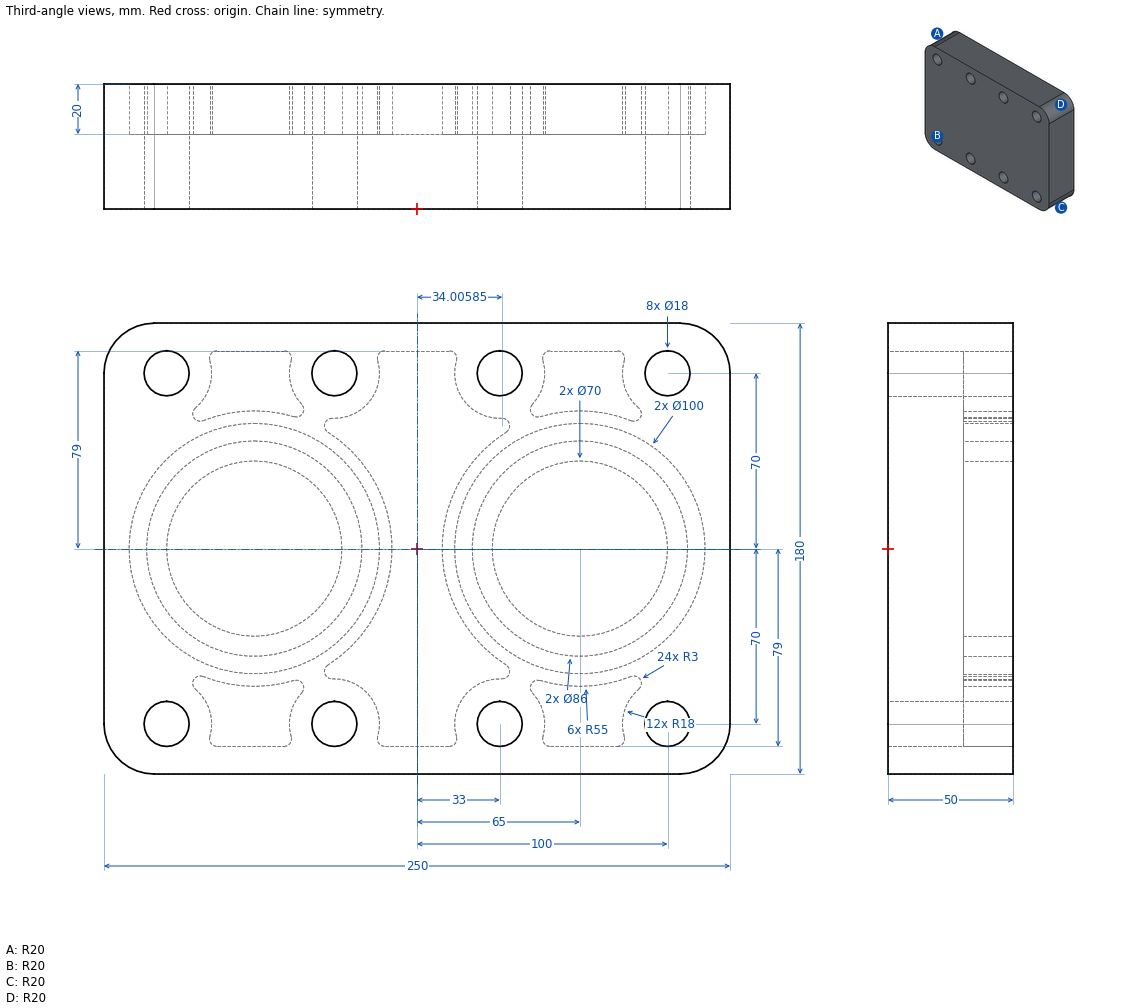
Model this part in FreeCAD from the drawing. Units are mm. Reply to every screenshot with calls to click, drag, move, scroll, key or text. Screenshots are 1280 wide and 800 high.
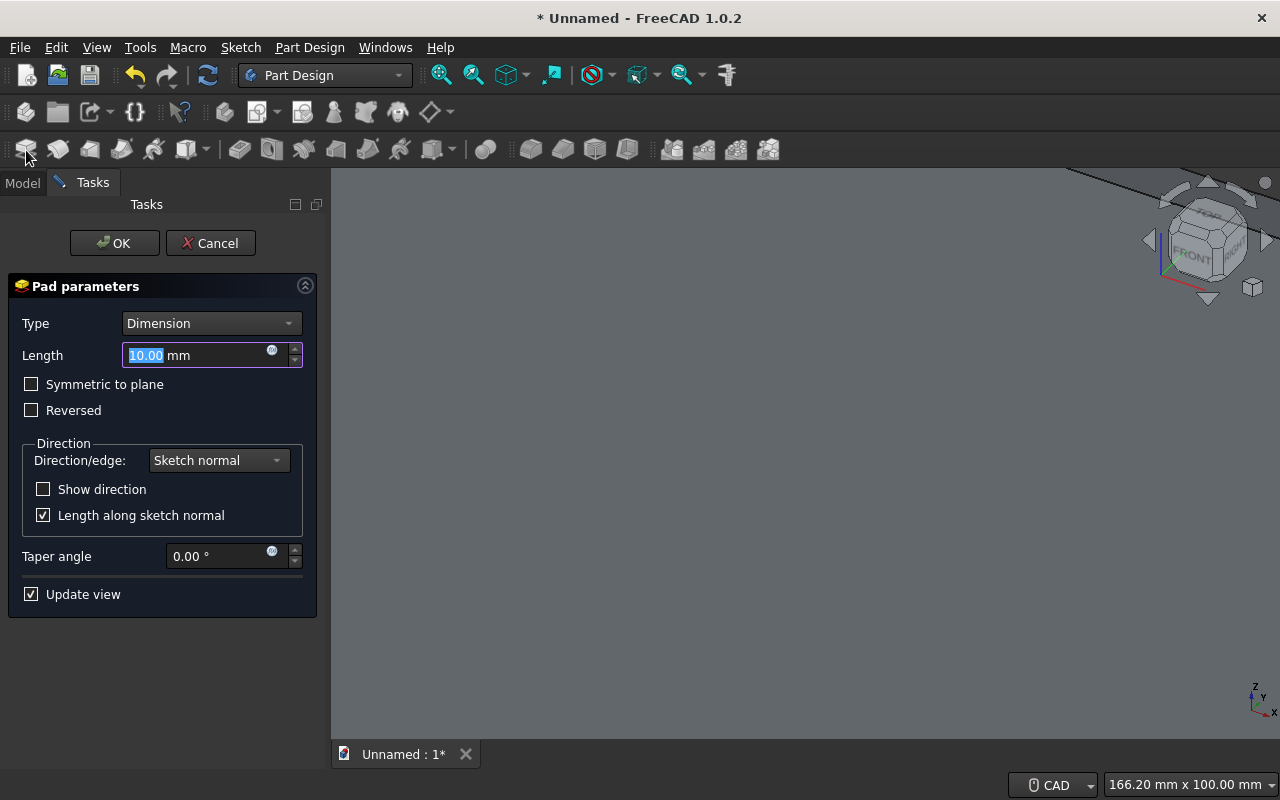
text(50)
key(Tab)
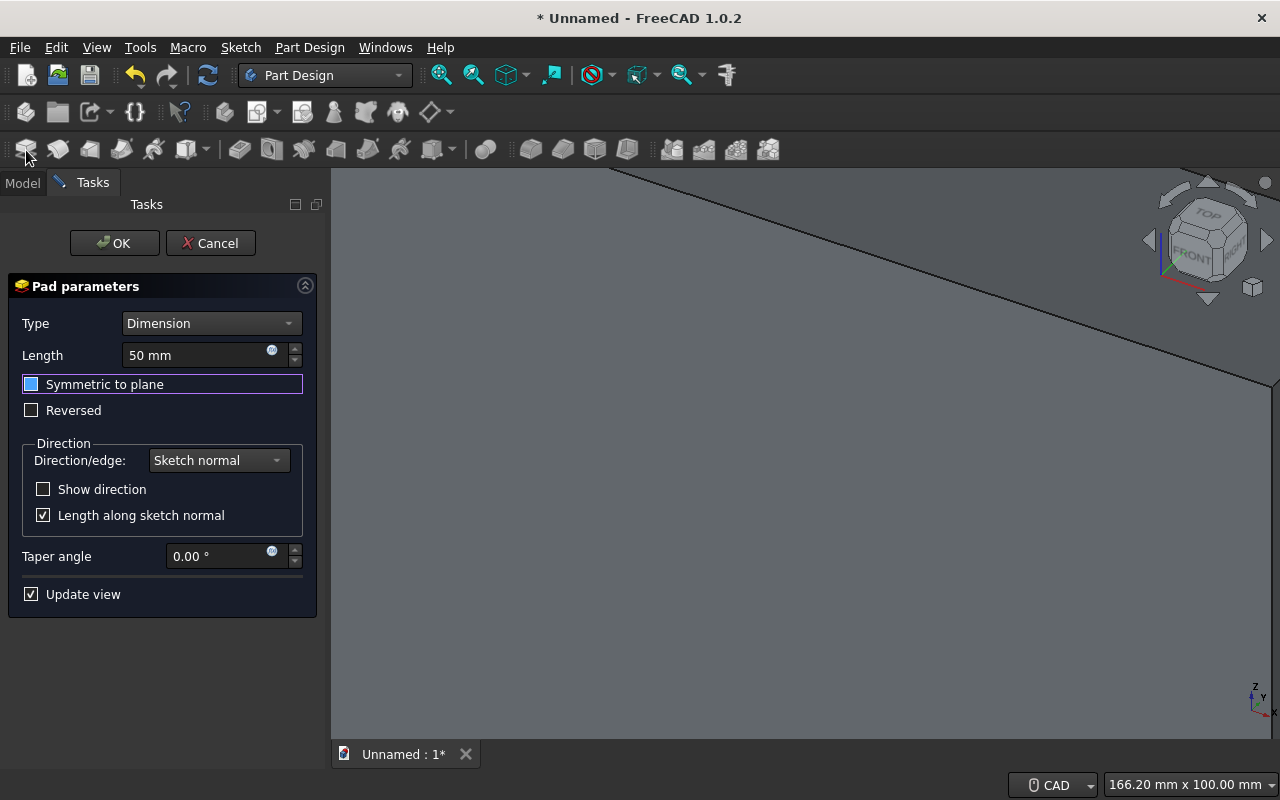
click(30, 410)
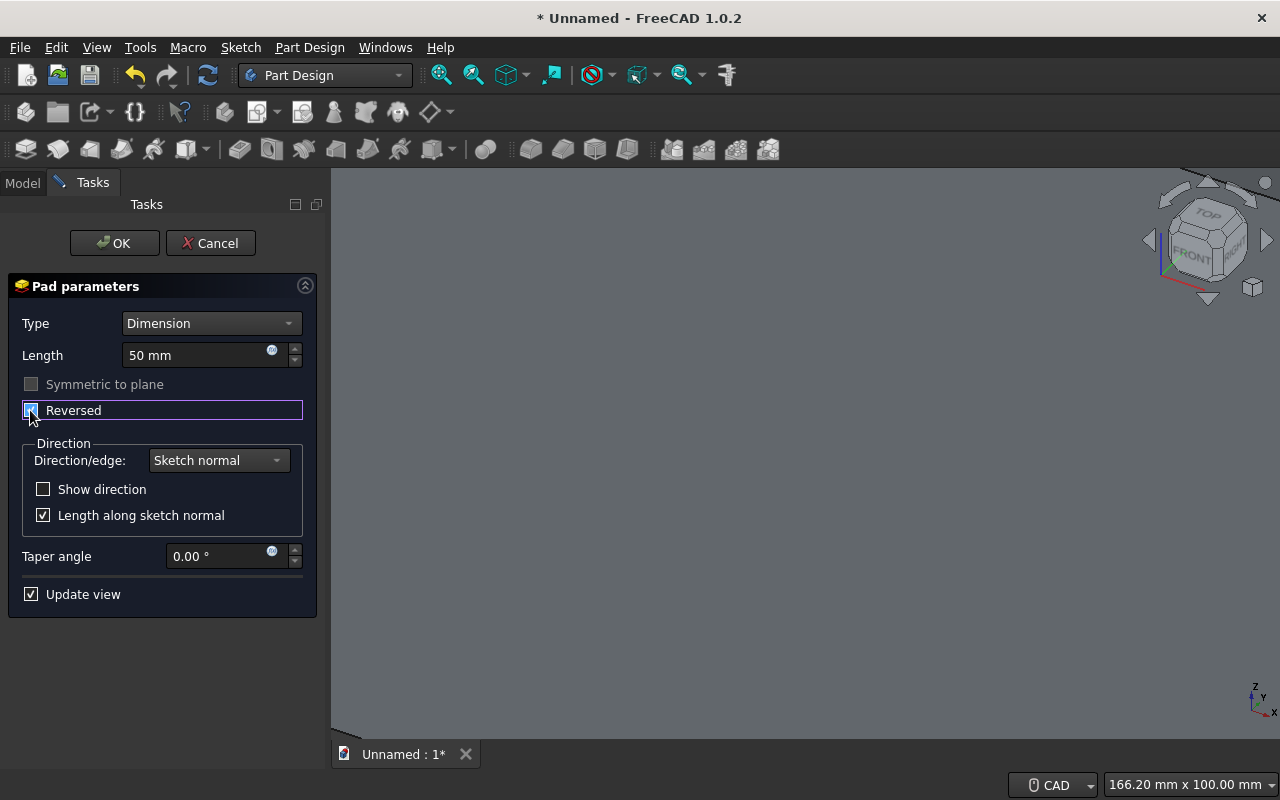
click(115, 243)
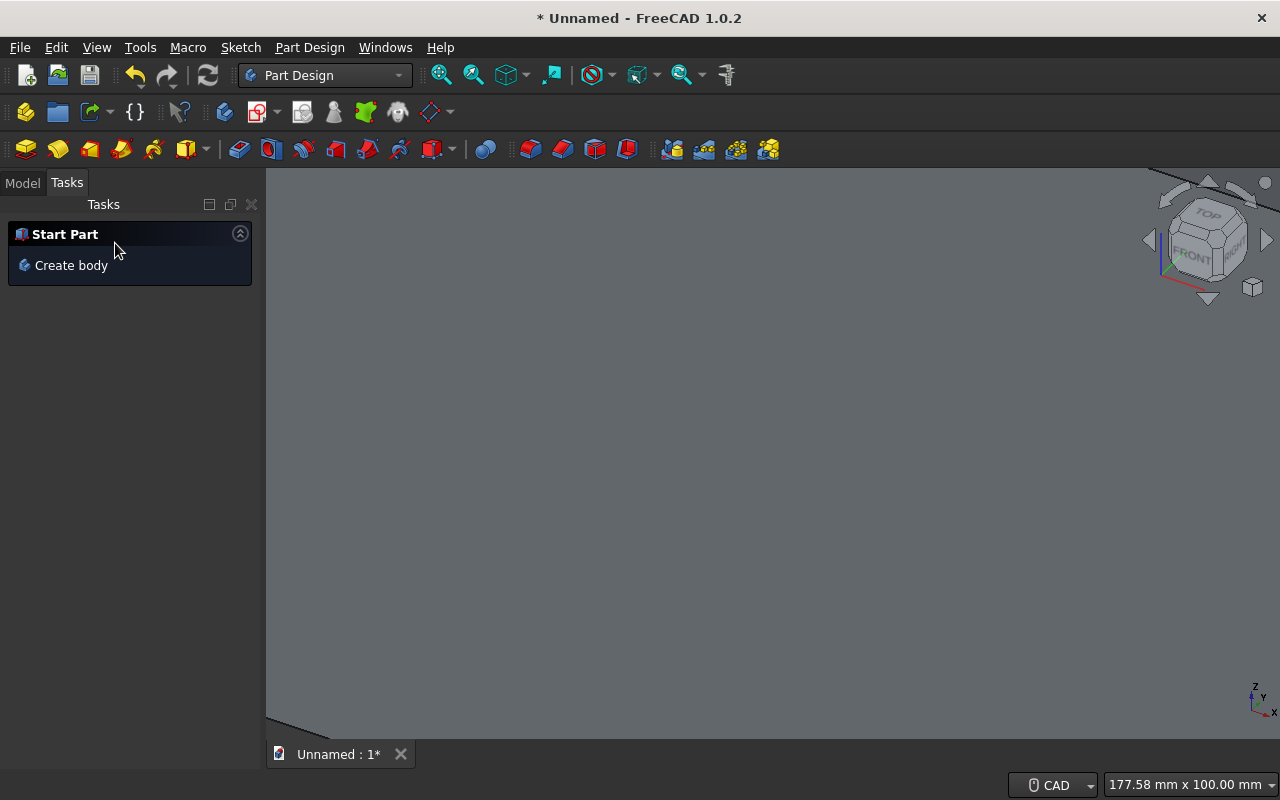
click(442, 76)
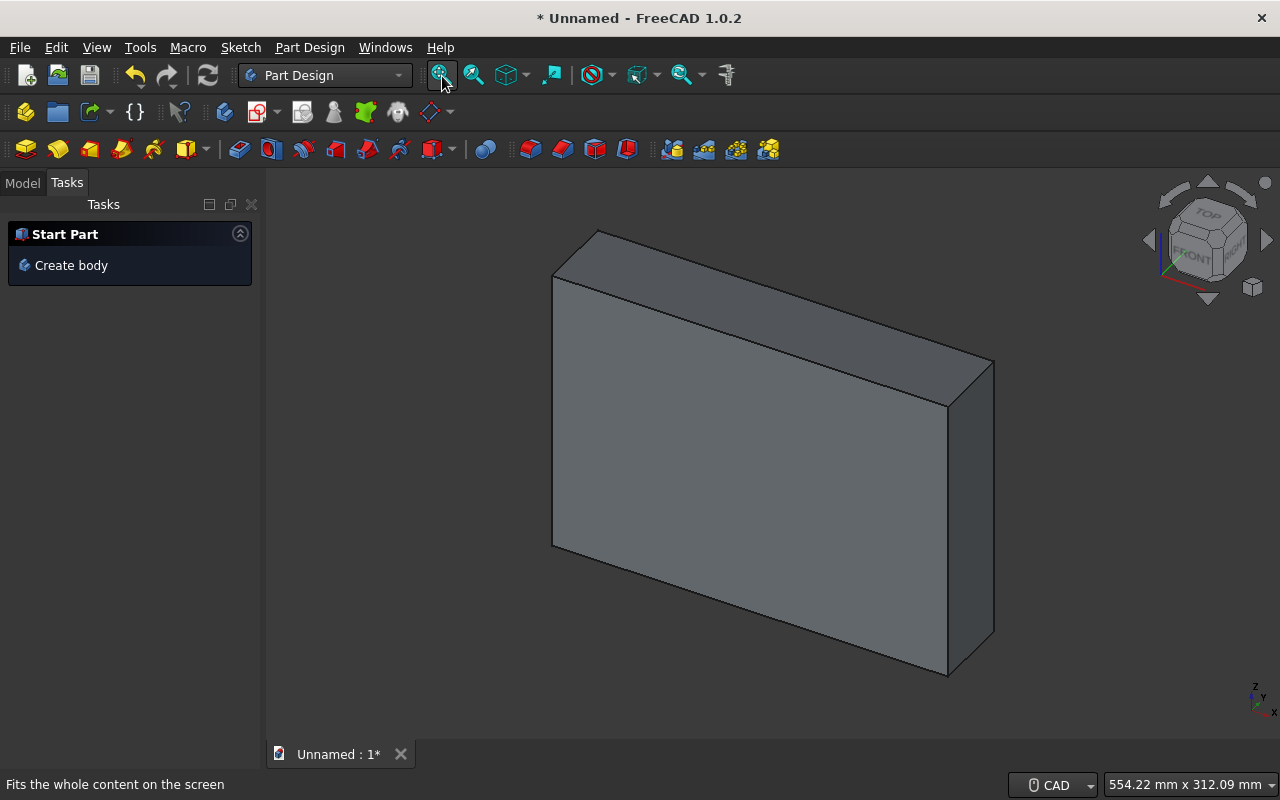
key(4)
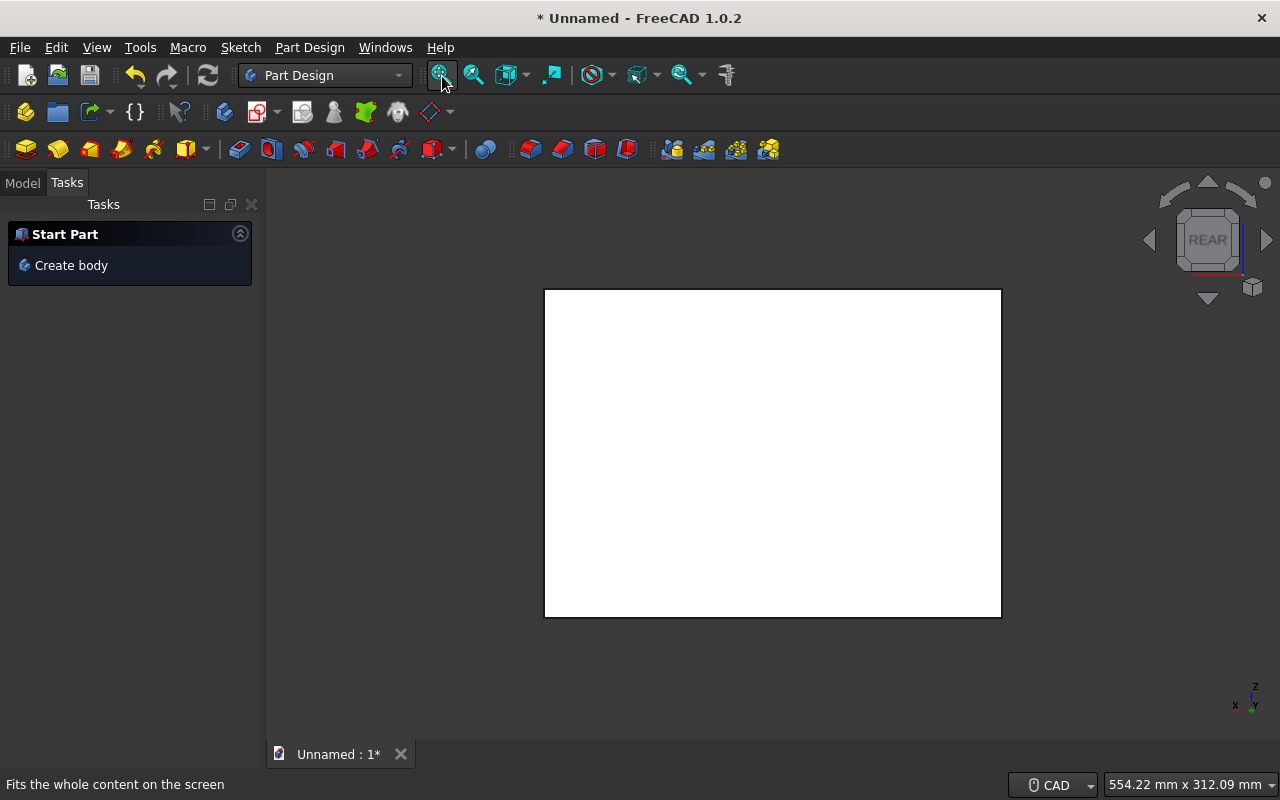
click(773, 453)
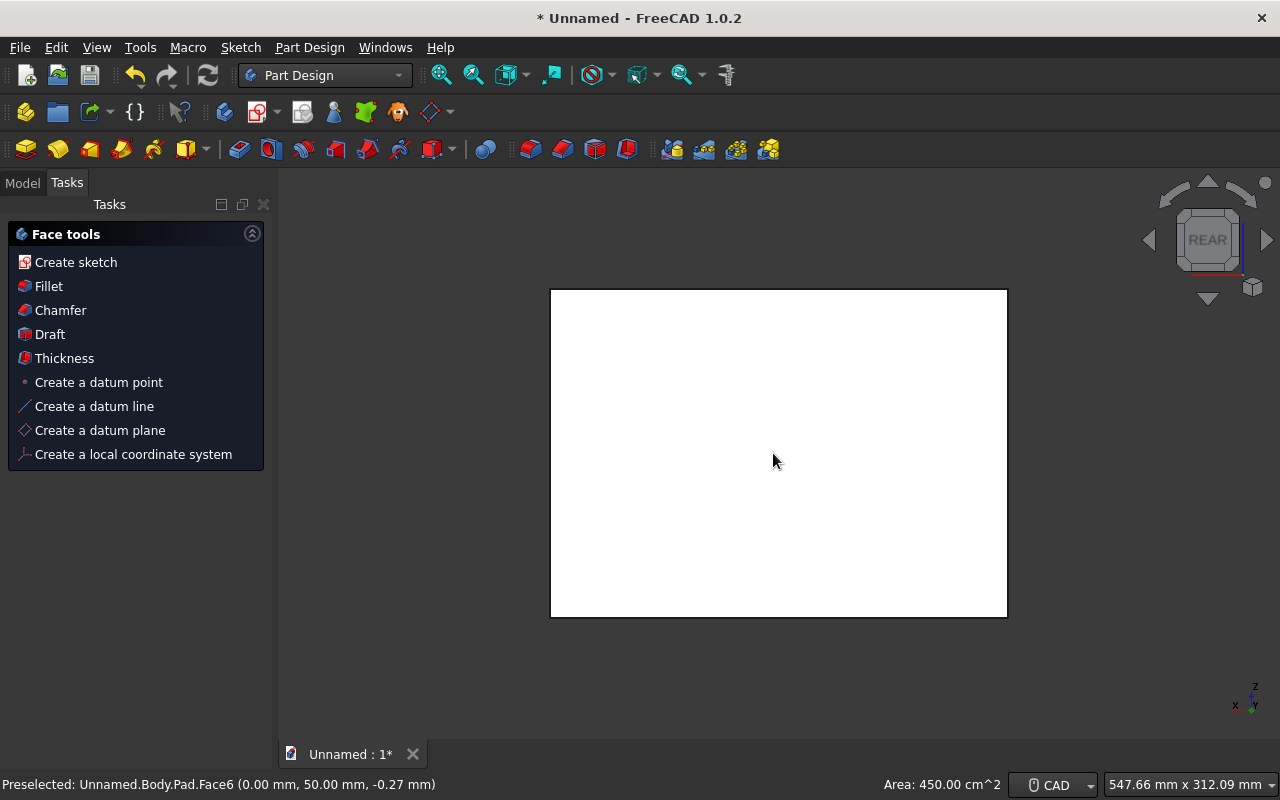
click(258, 112)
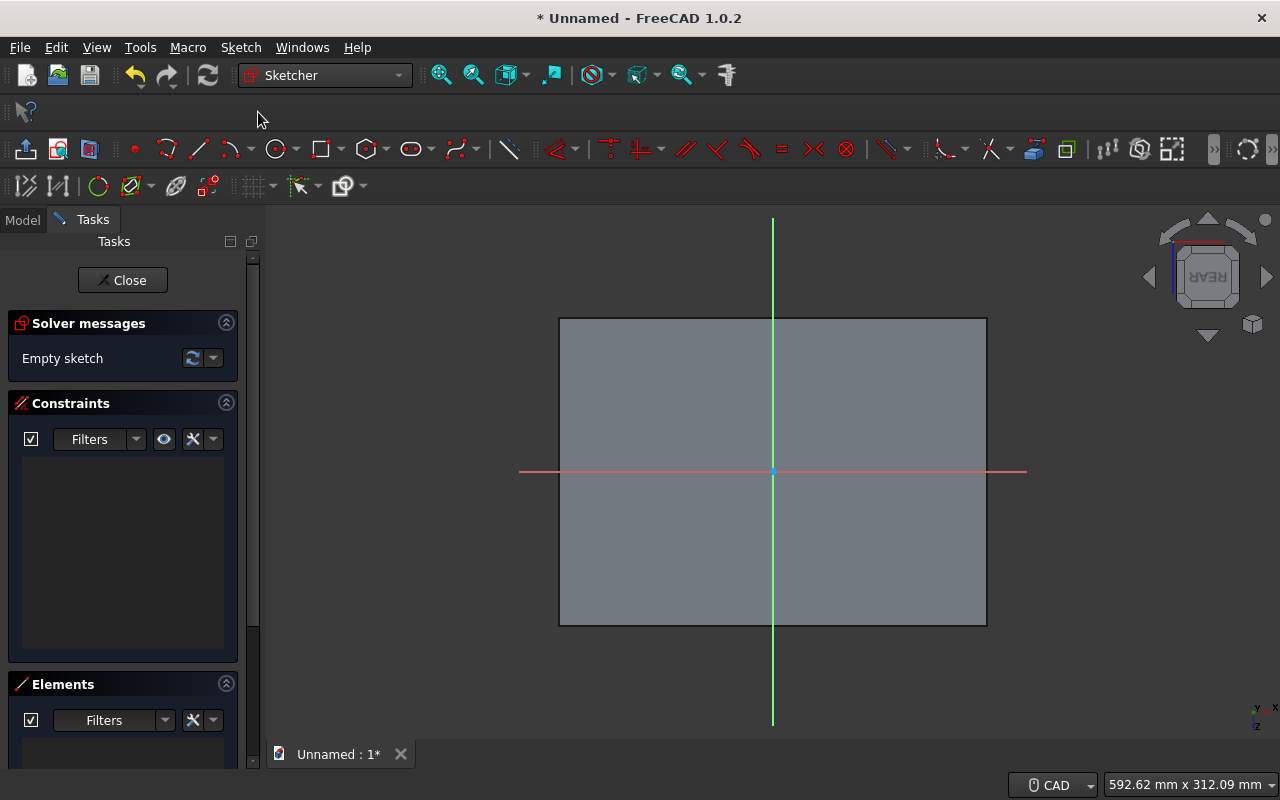
click(200, 150)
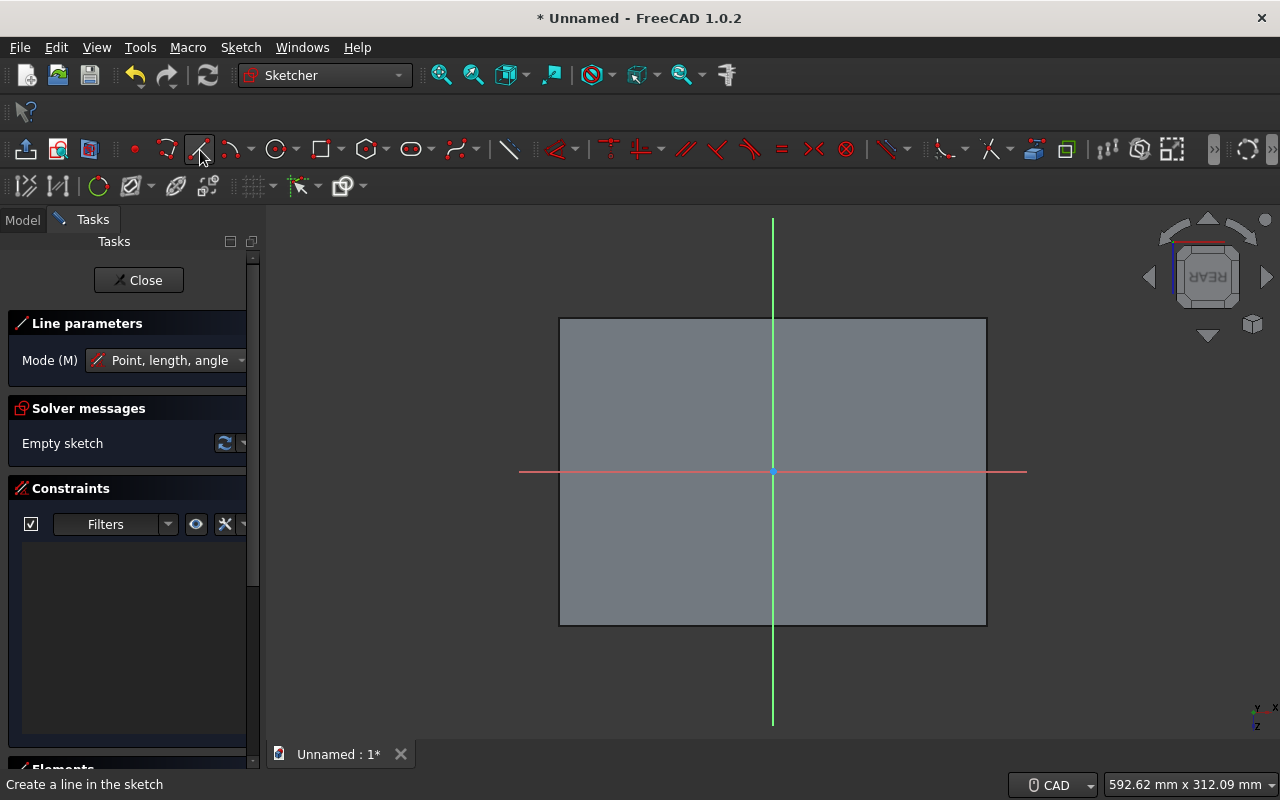
click(910, 337)
click(864, 337)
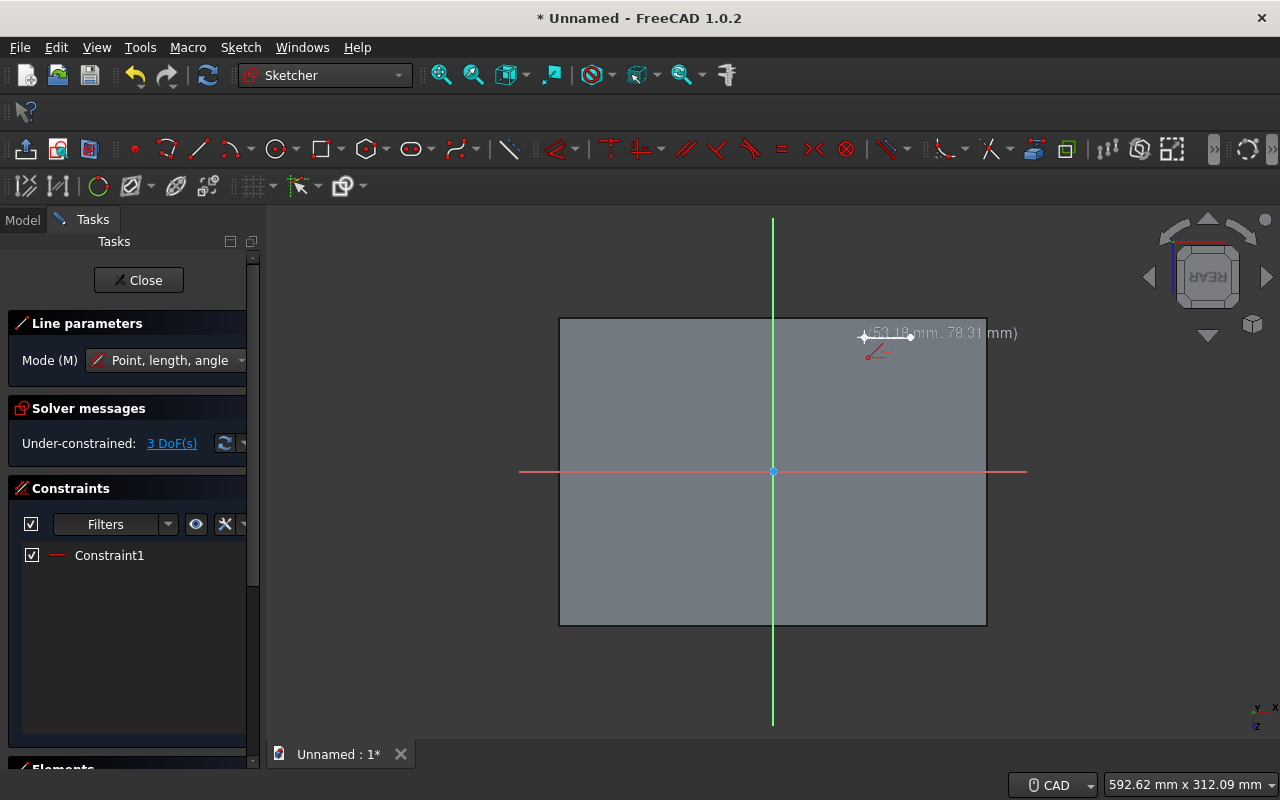
key(g)
key(3)
key(a)